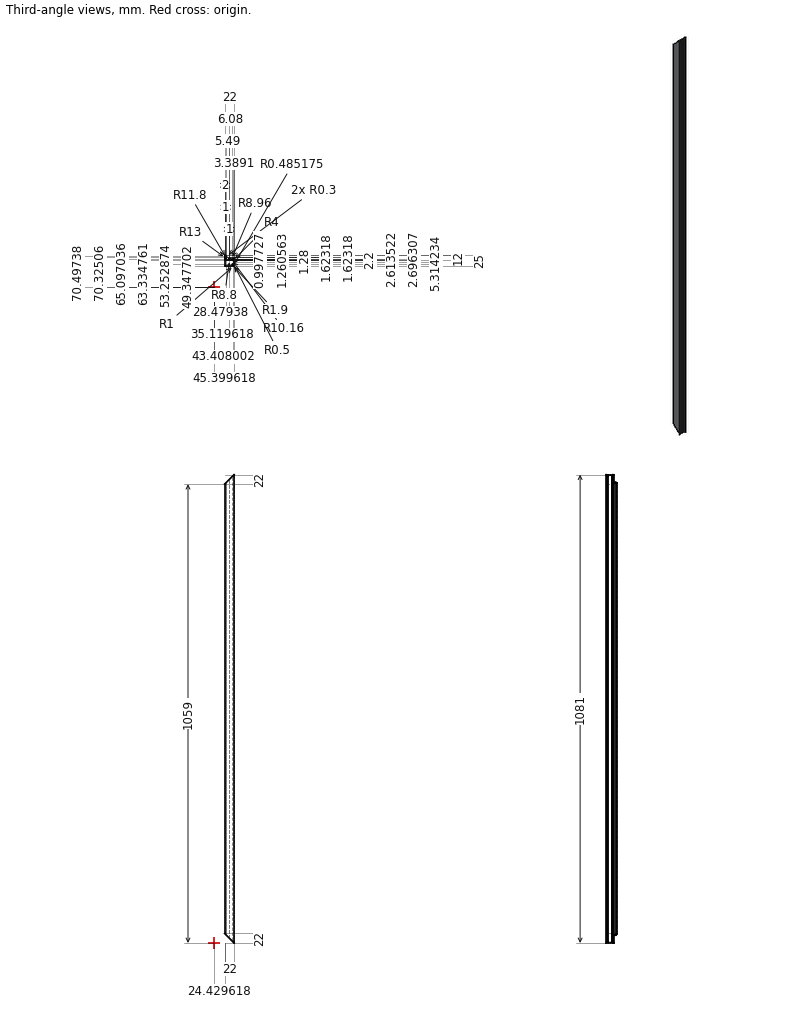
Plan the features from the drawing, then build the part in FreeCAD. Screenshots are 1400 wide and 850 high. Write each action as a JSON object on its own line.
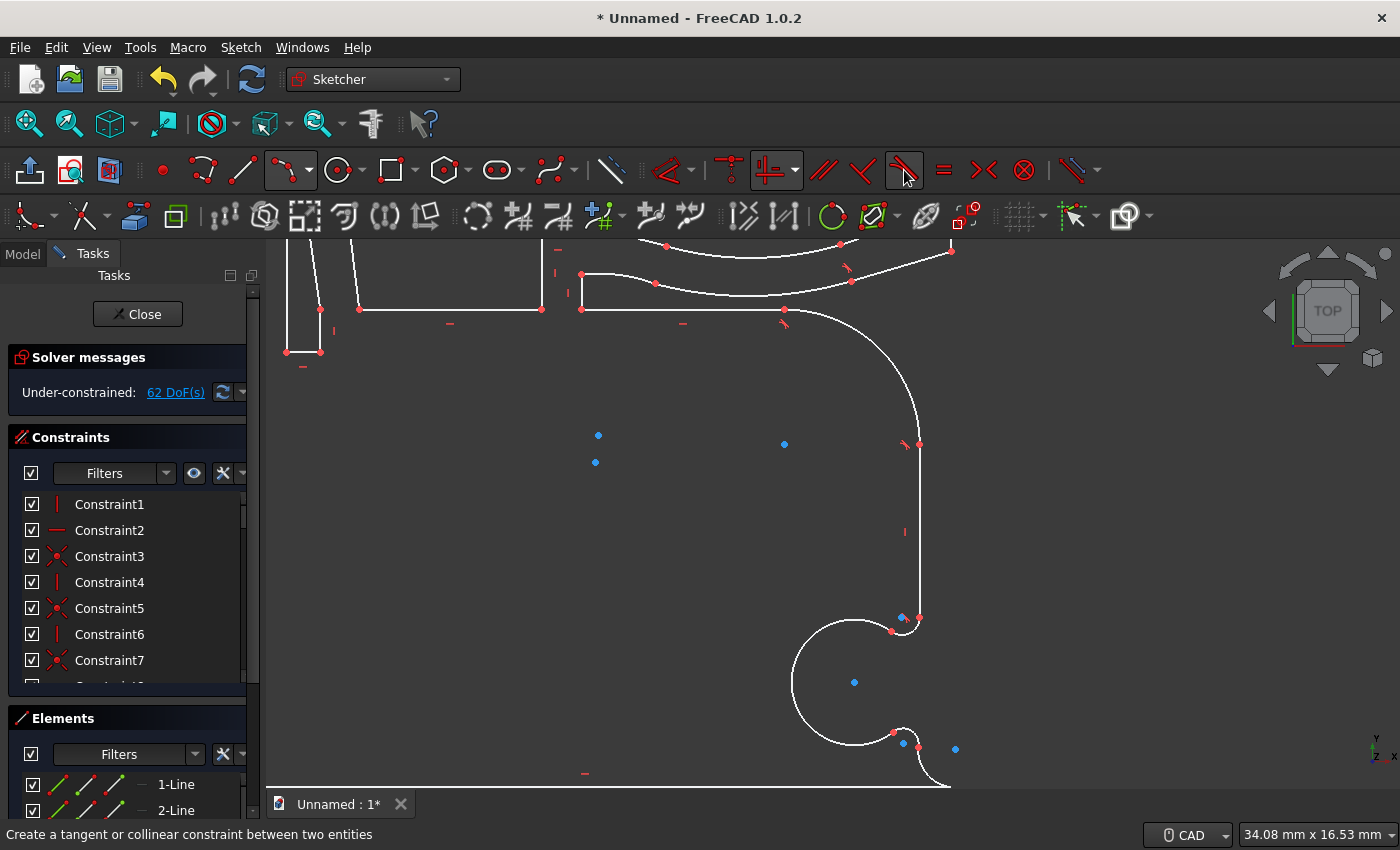
{"action": "scroll", "coordinate": [910, 633], "scroll_direction": "down", "scroll_amount": 4}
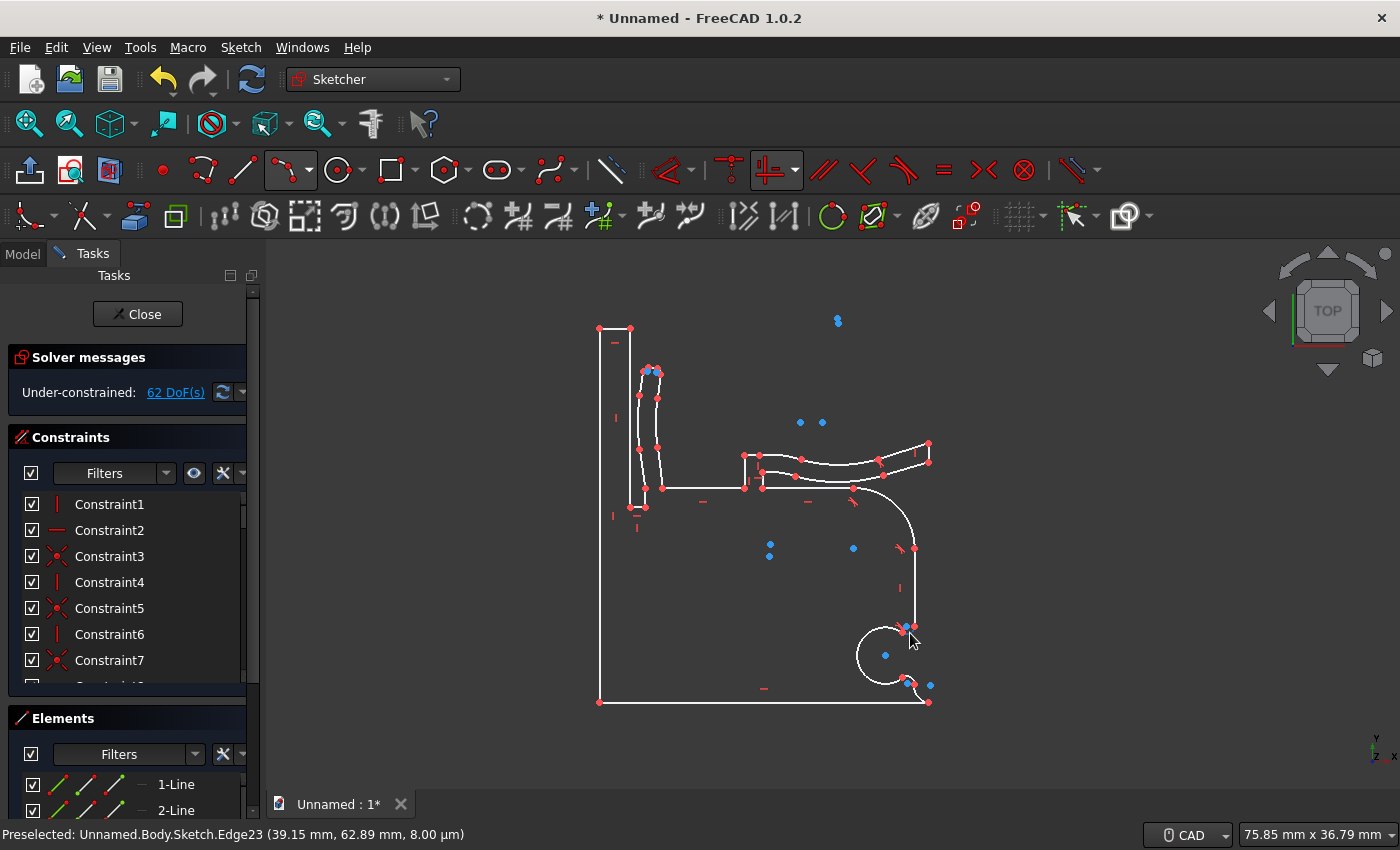
{"action": "left_click", "coordinate": [894, 454]}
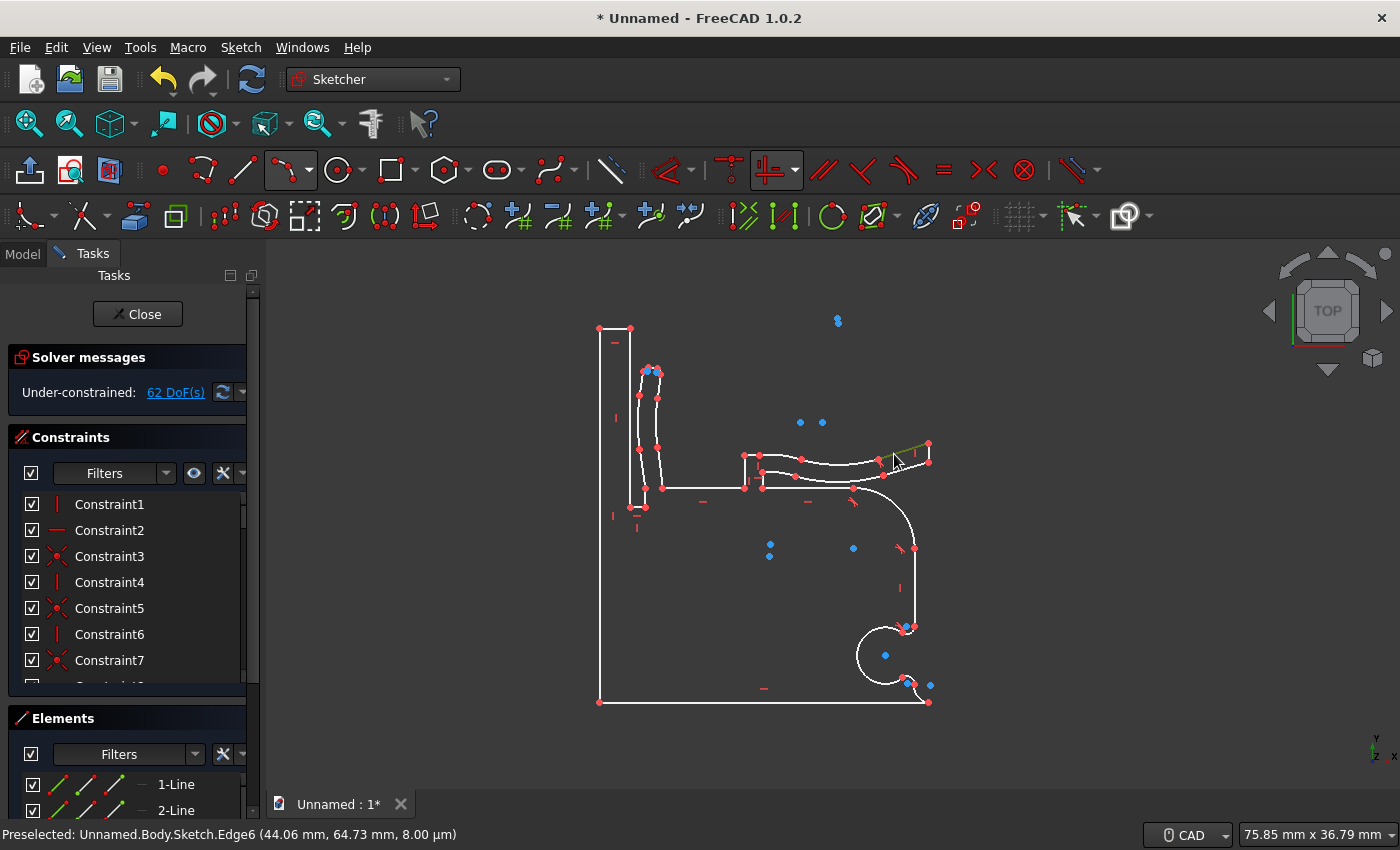
{"action": "left_click", "coordinate": [824, 464]}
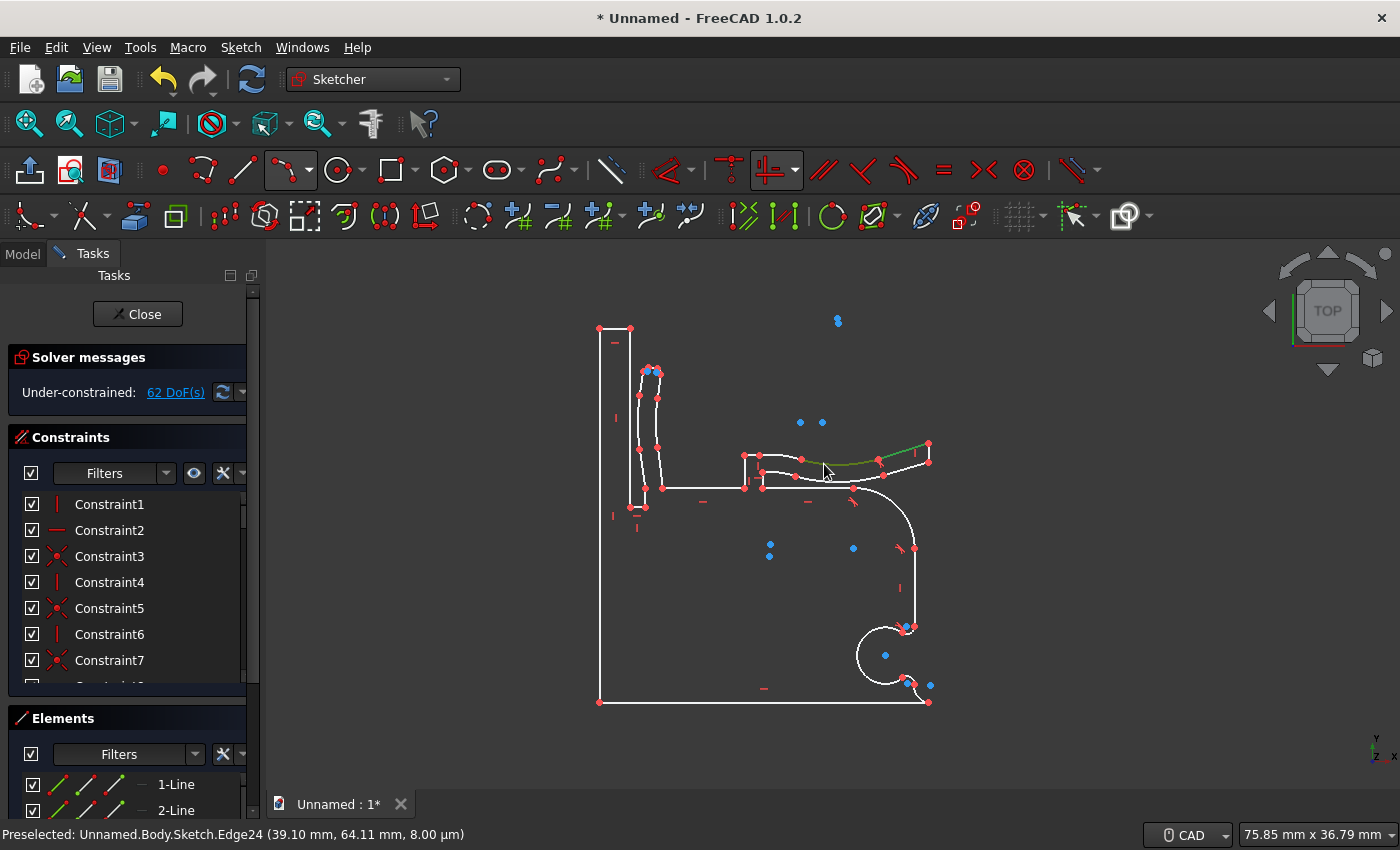
{"action": "left_click", "coordinate": [904, 170]}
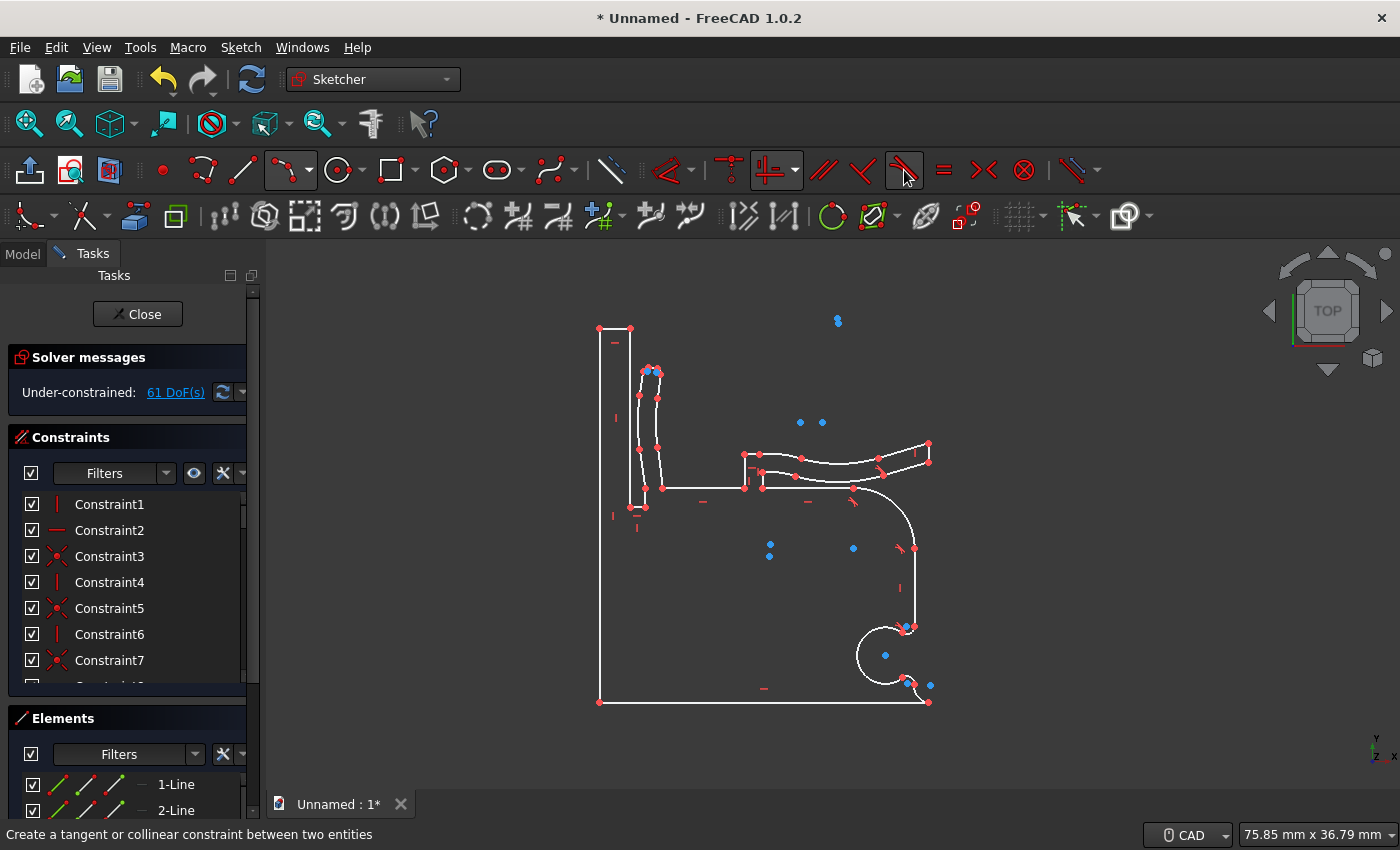
{"action": "scroll", "coordinate": [752, 454], "scroll_direction": "up", "scroll_amount": 4}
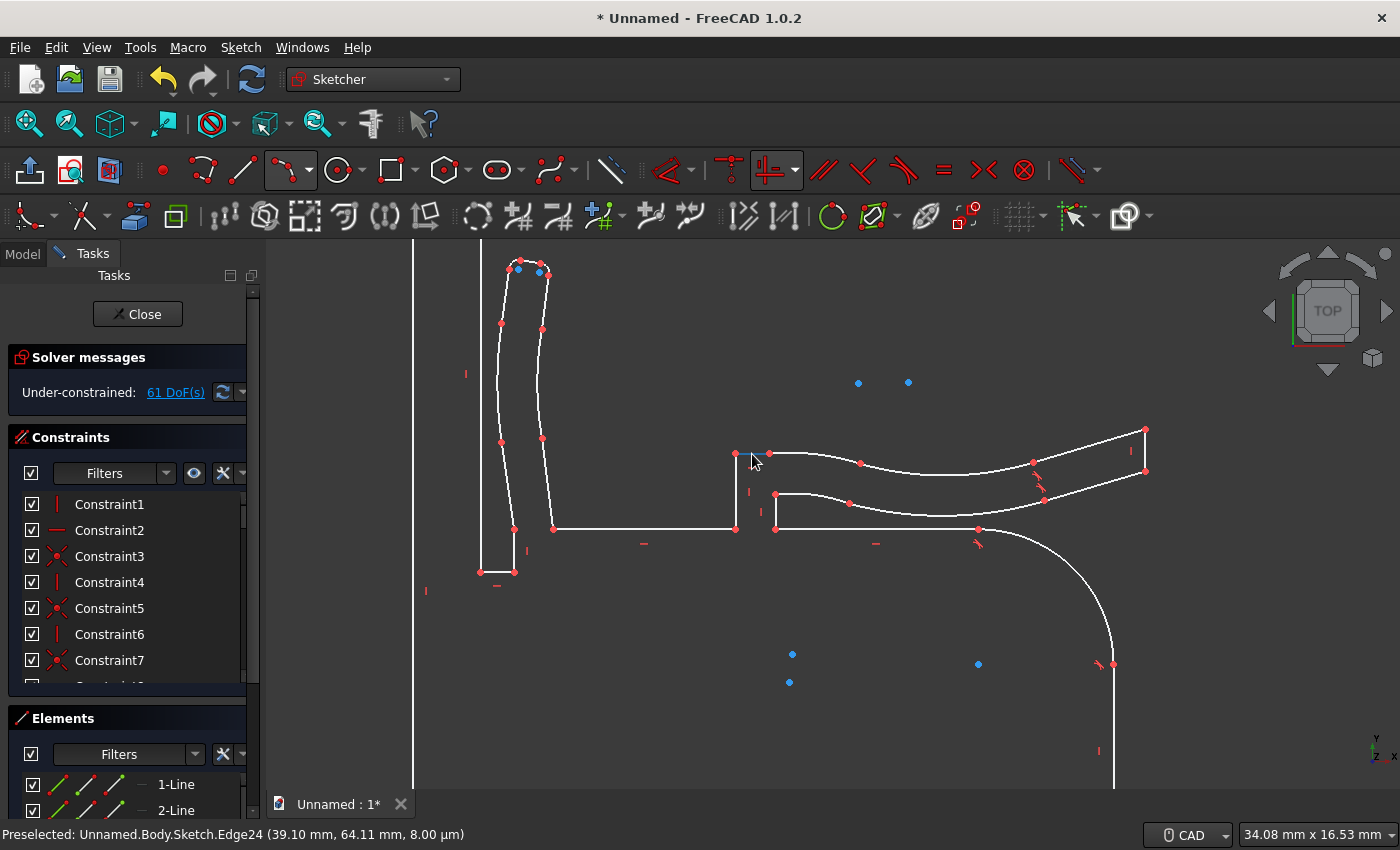
{"action": "left_click", "coordinate": [752, 454]}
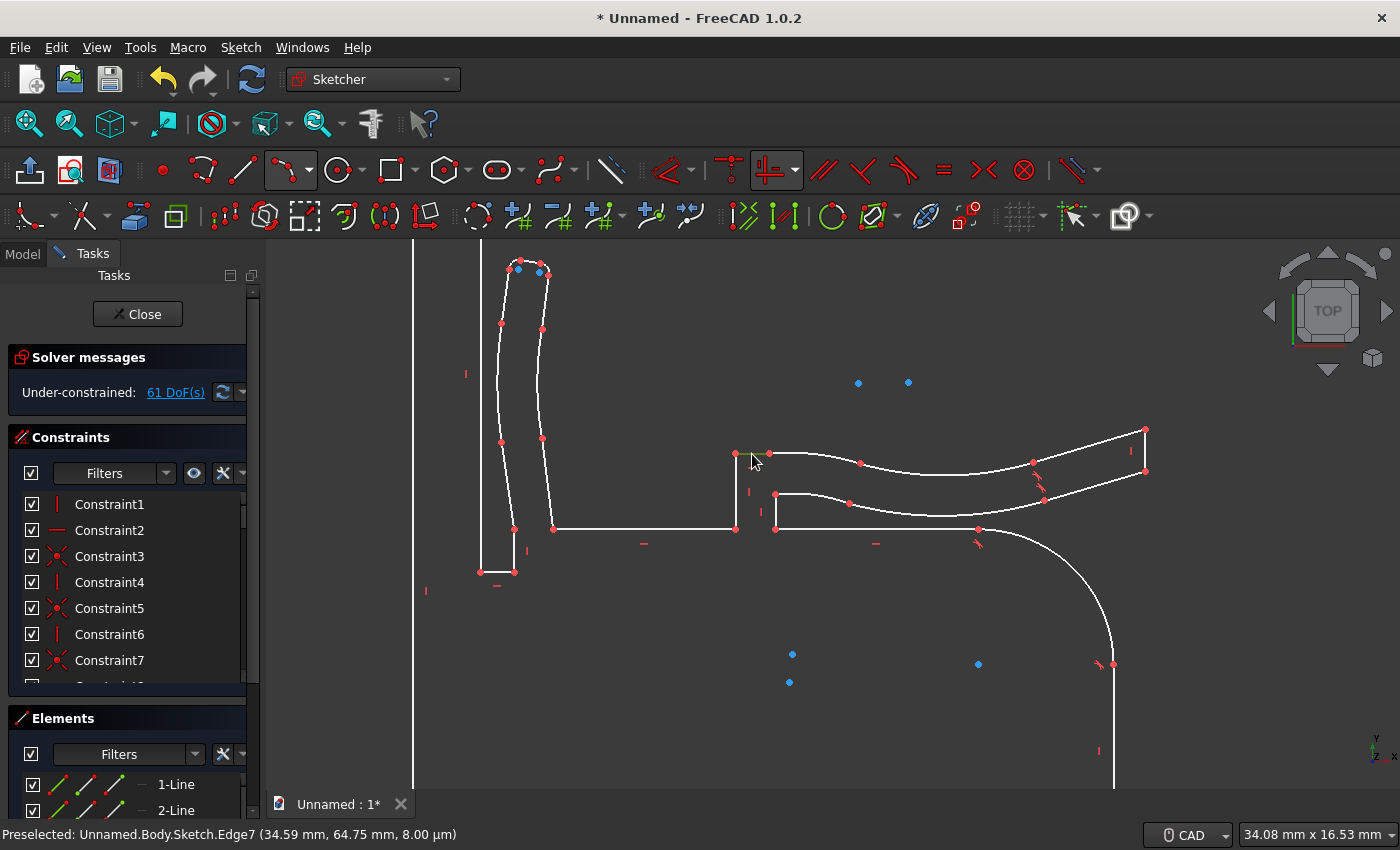
{"action": "left_click", "coordinate": [834, 457]}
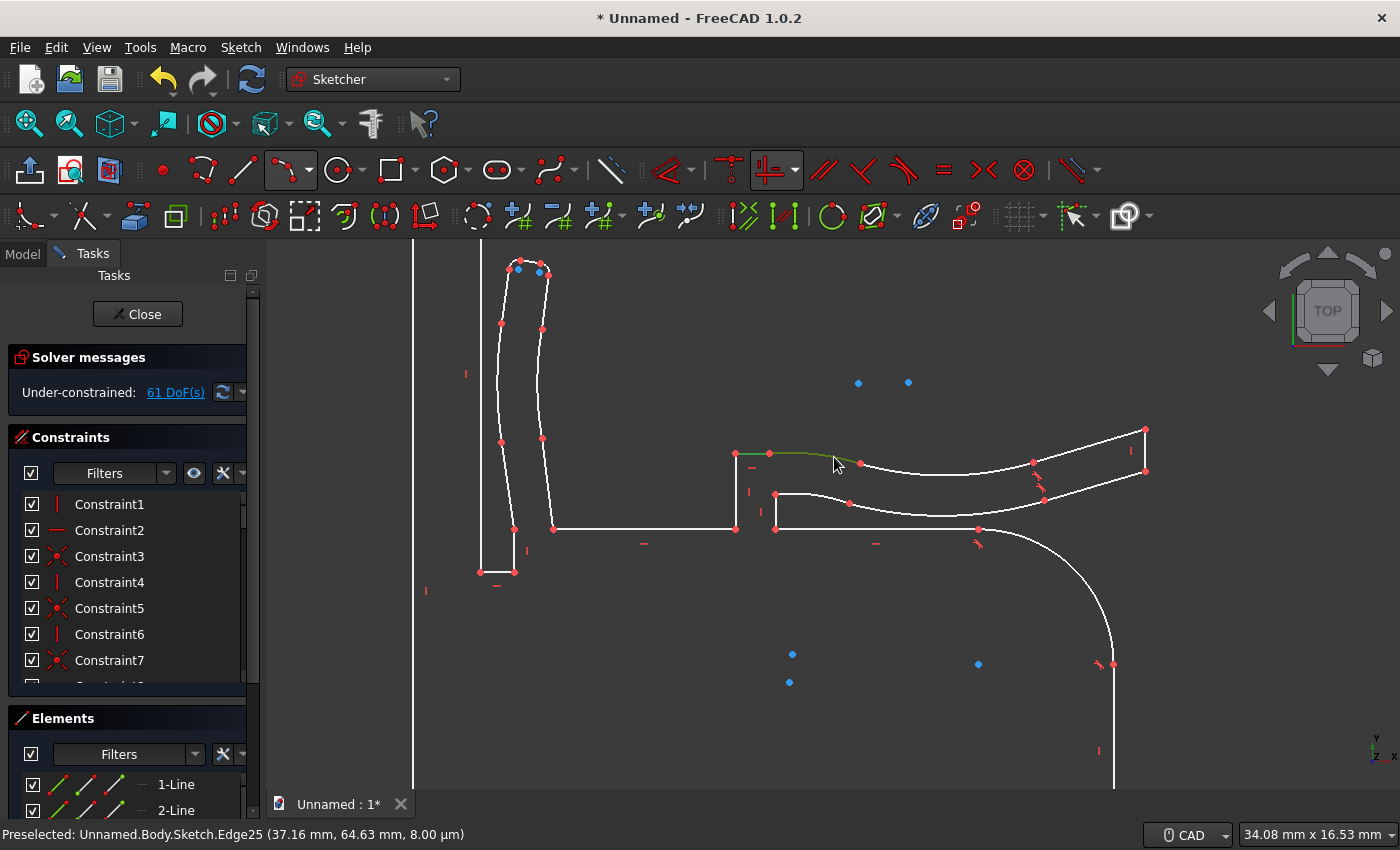
{"action": "left_click", "coordinate": [904, 170]}